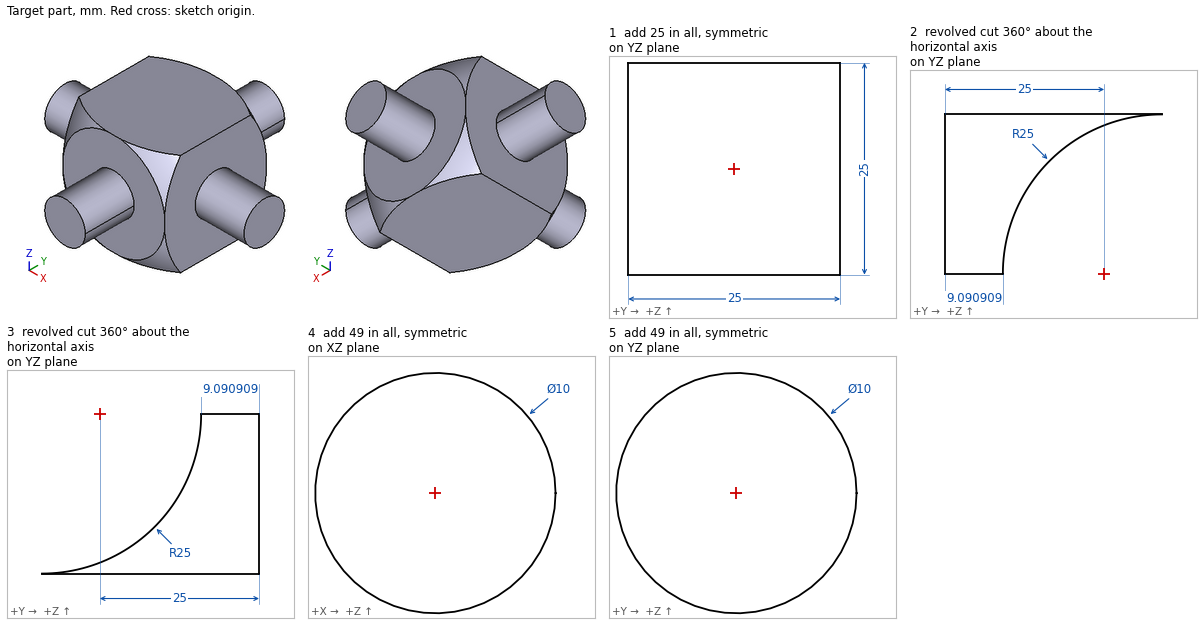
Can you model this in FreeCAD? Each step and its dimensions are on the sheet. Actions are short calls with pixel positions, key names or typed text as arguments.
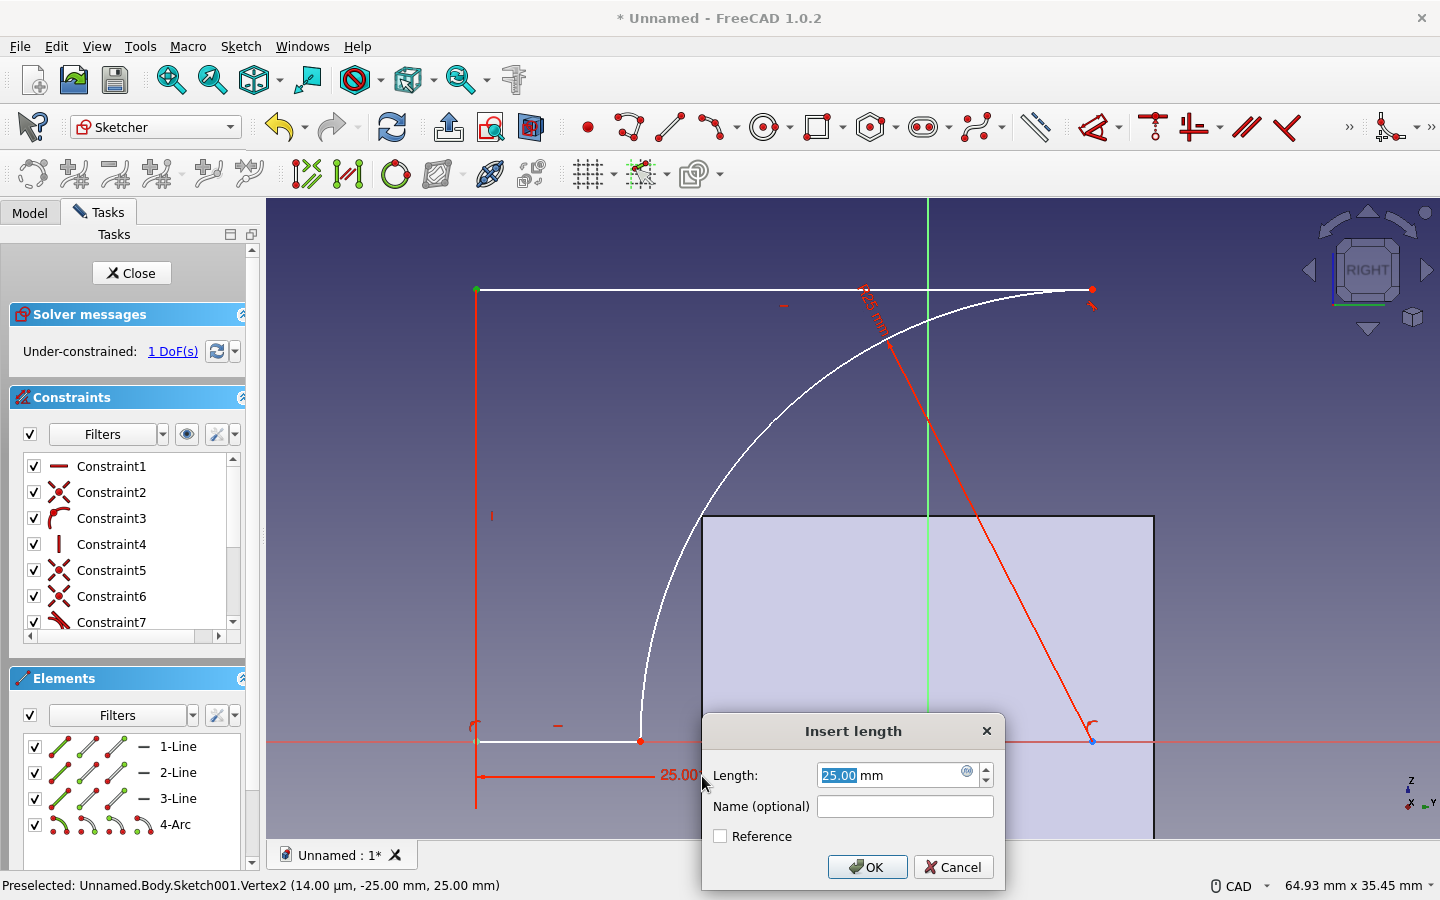
text(25)
key(Return)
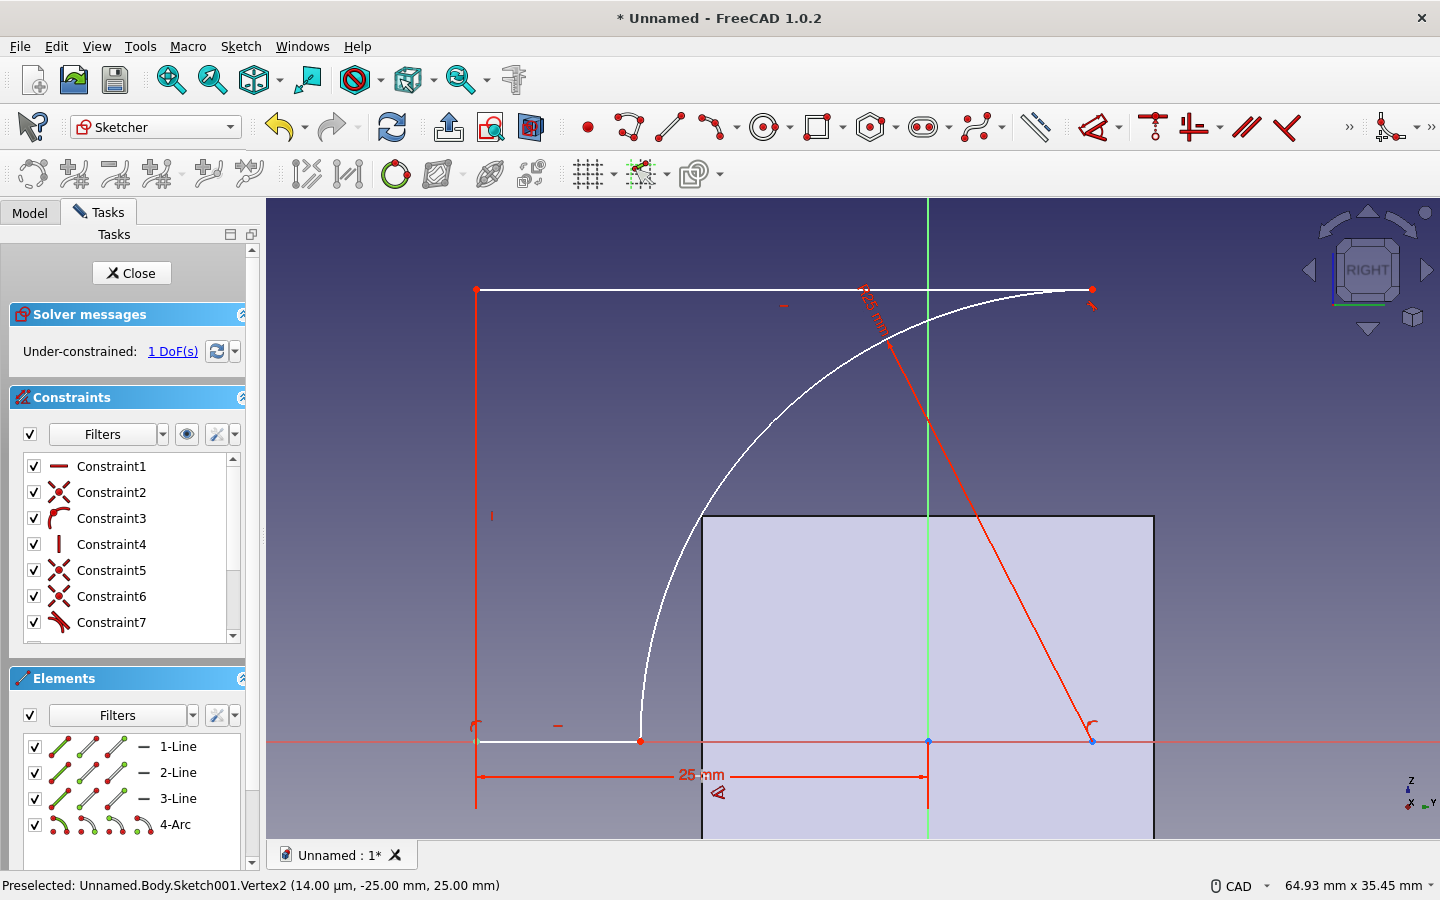
click(525, 742)
click(558, 776)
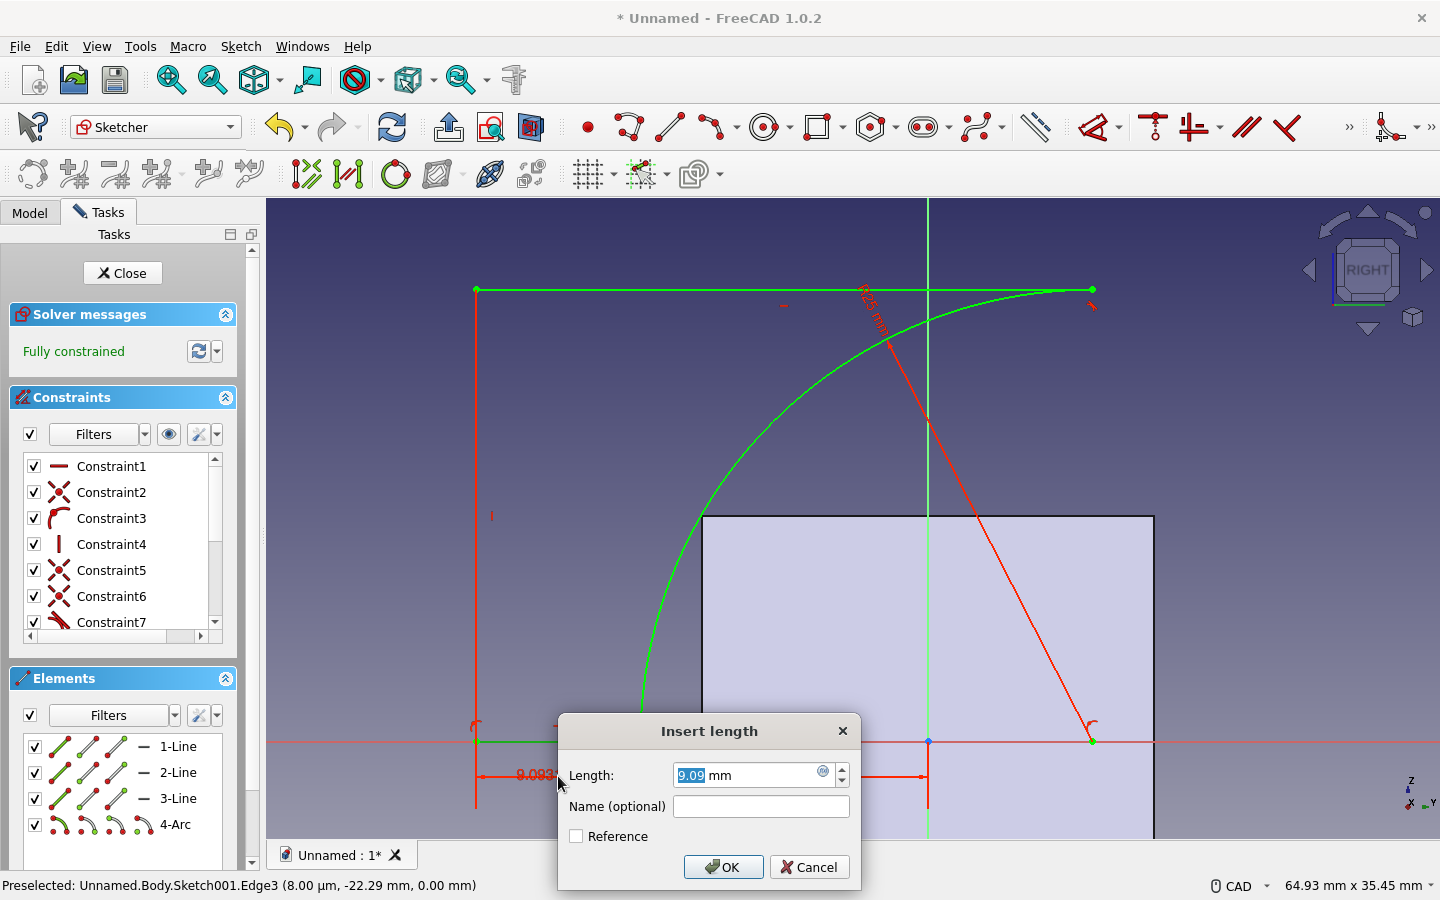
text(9.090909)
key(Return)
key(Escape)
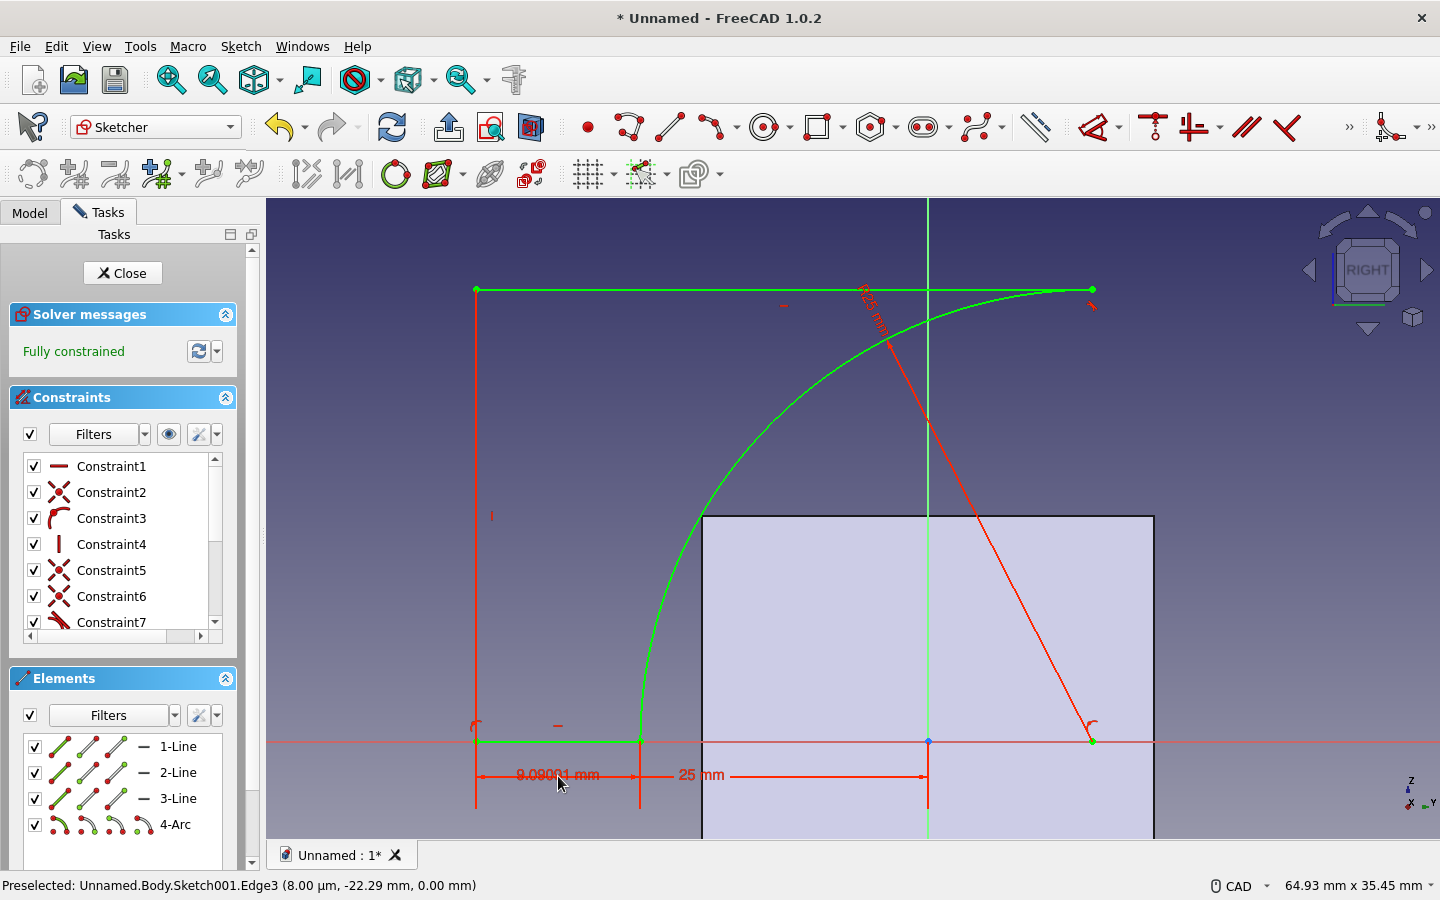
click(123, 273)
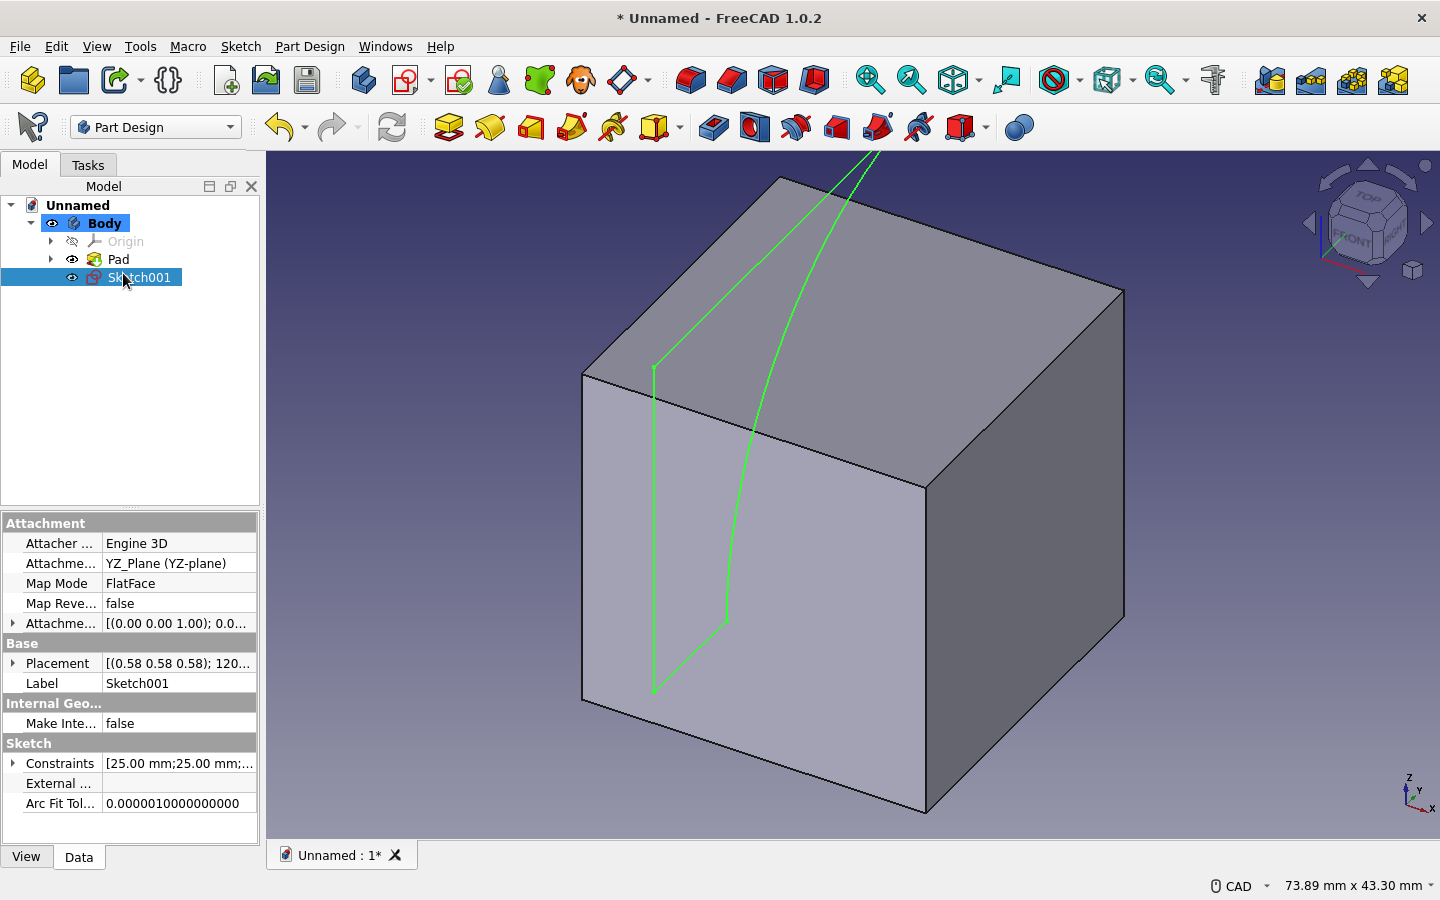
click(796, 128)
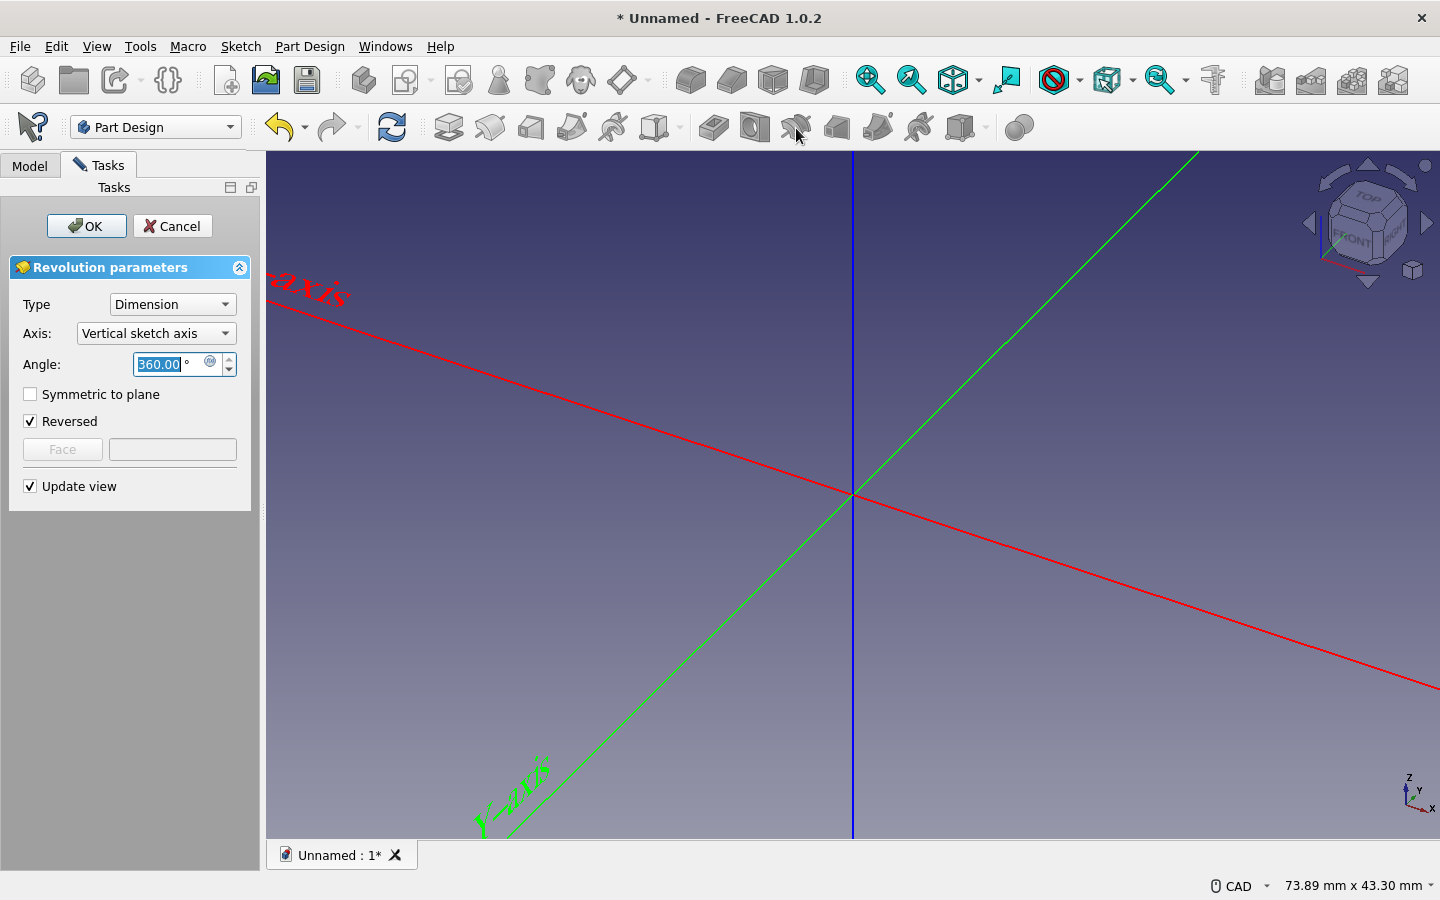
click(157, 334)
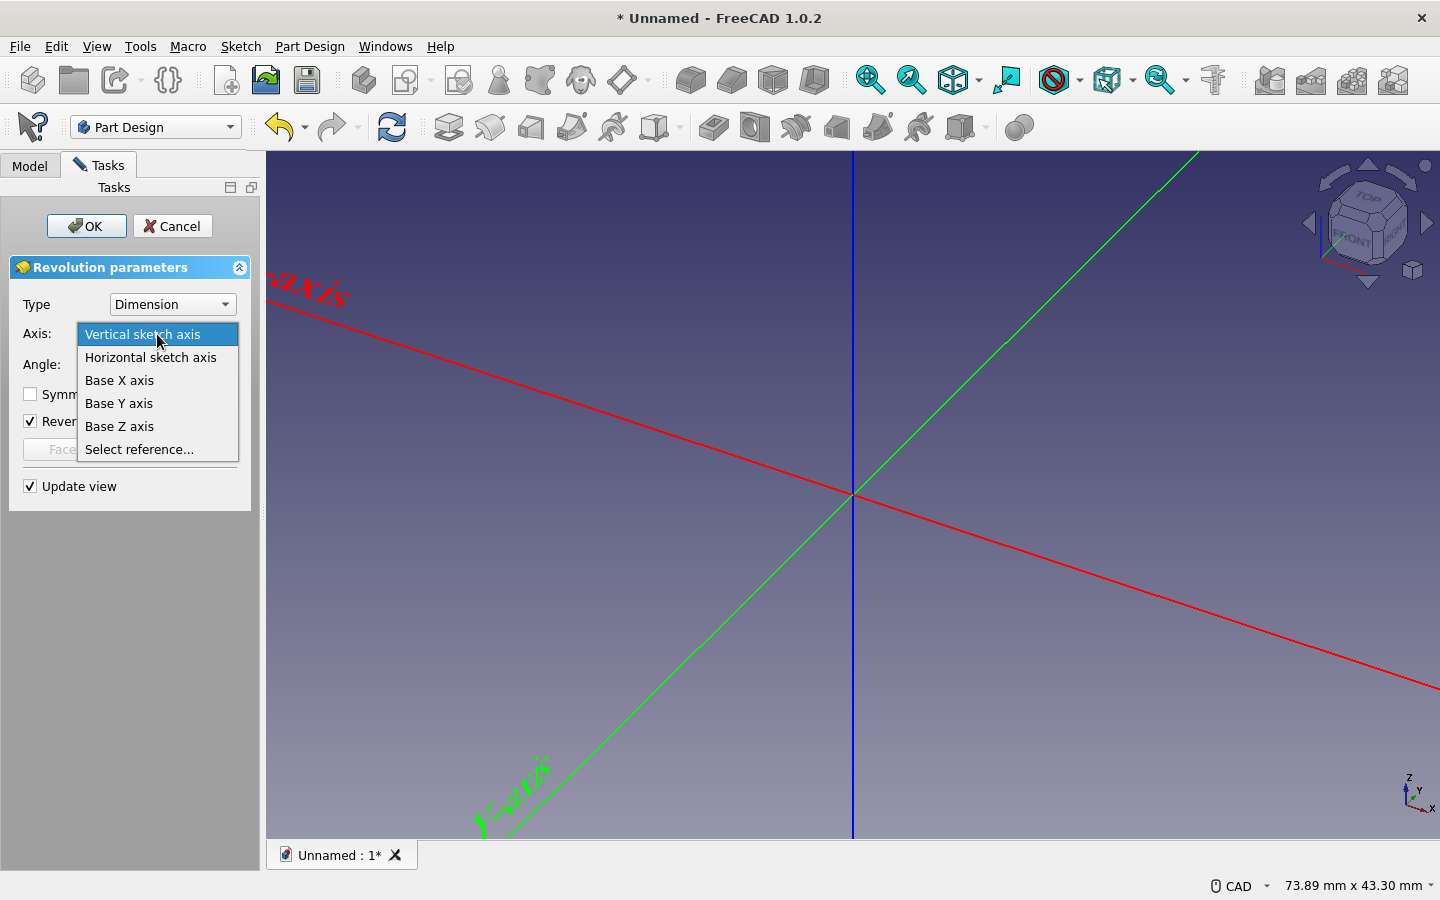
click(156, 358)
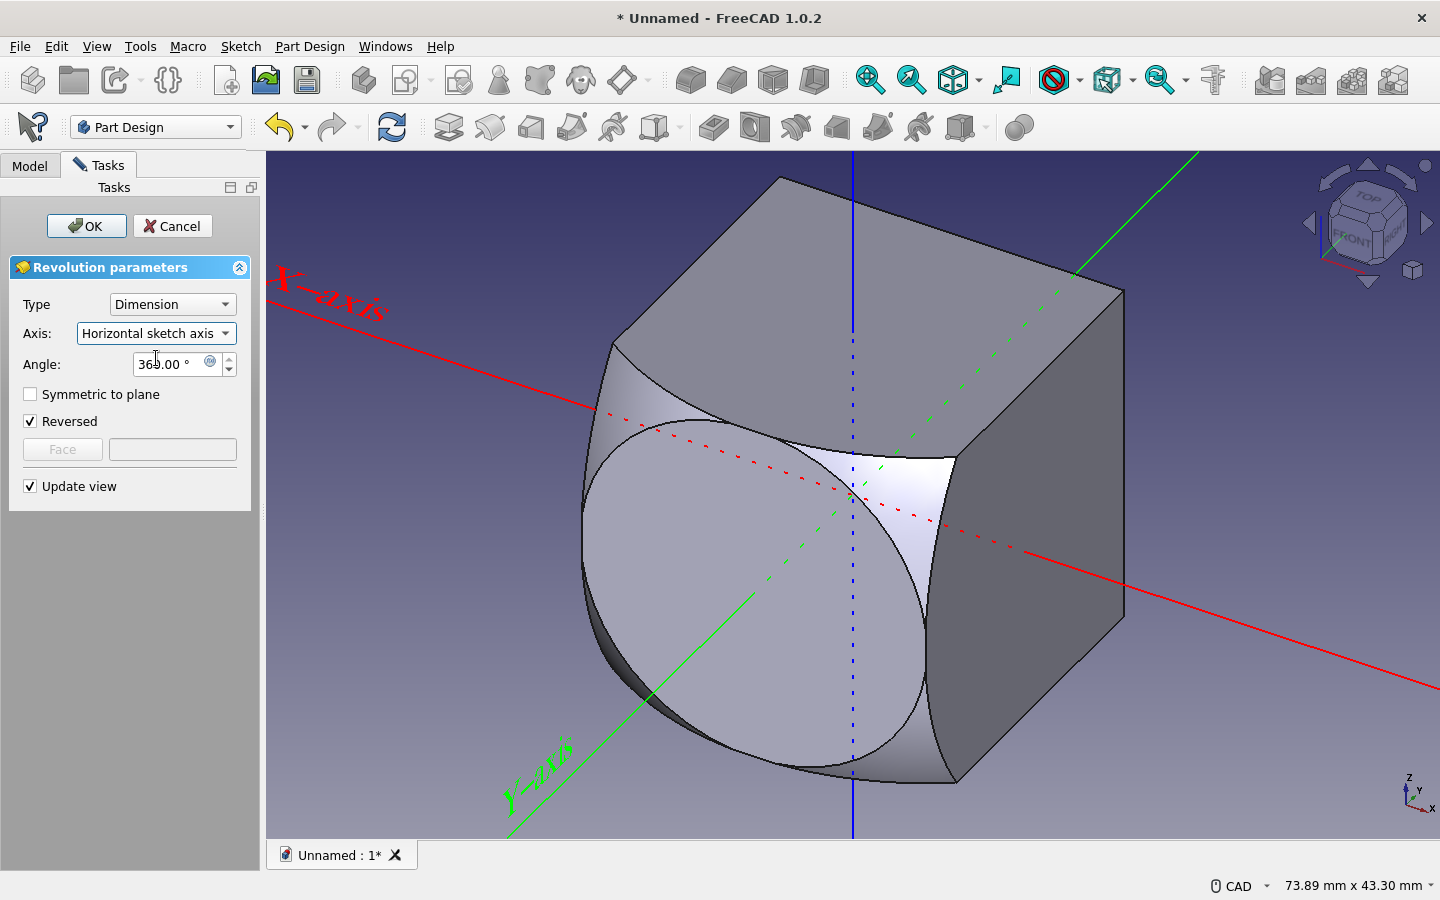
click(87, 226)